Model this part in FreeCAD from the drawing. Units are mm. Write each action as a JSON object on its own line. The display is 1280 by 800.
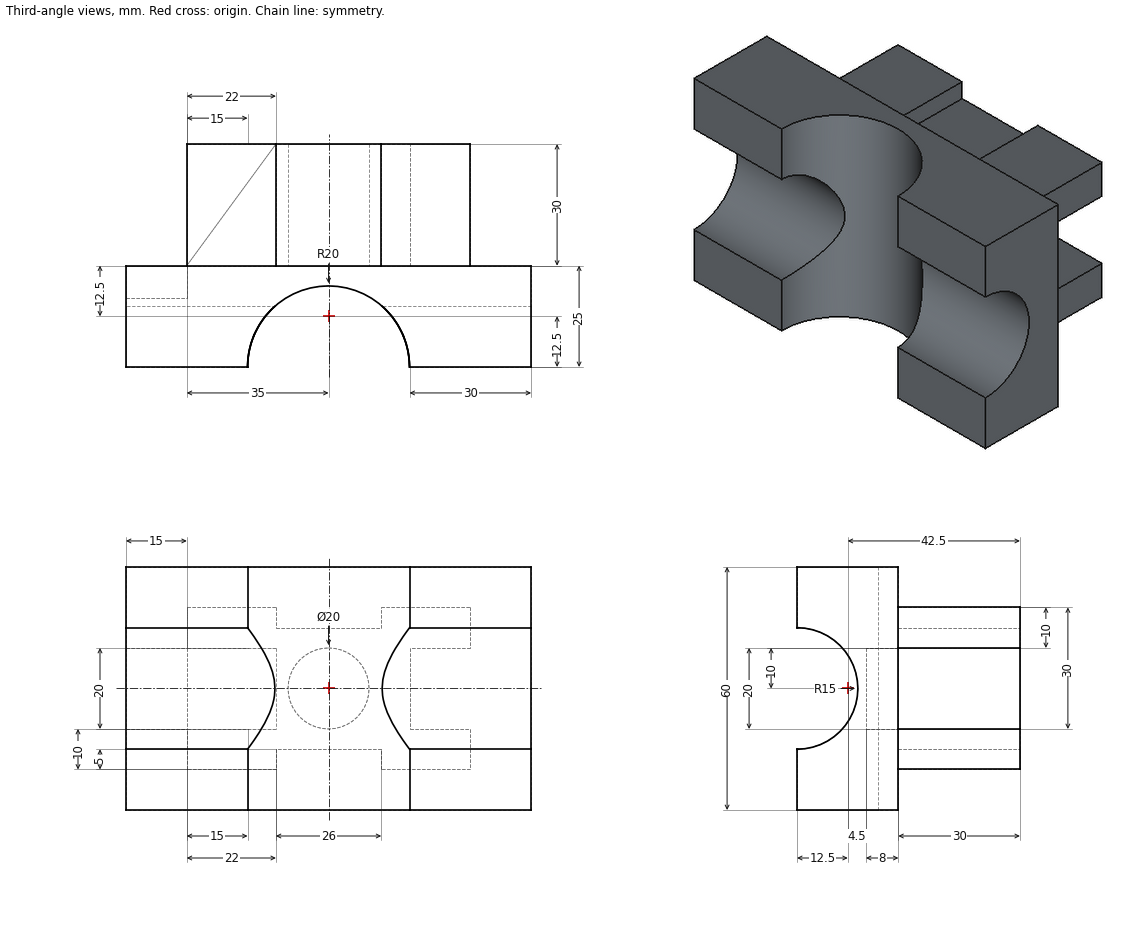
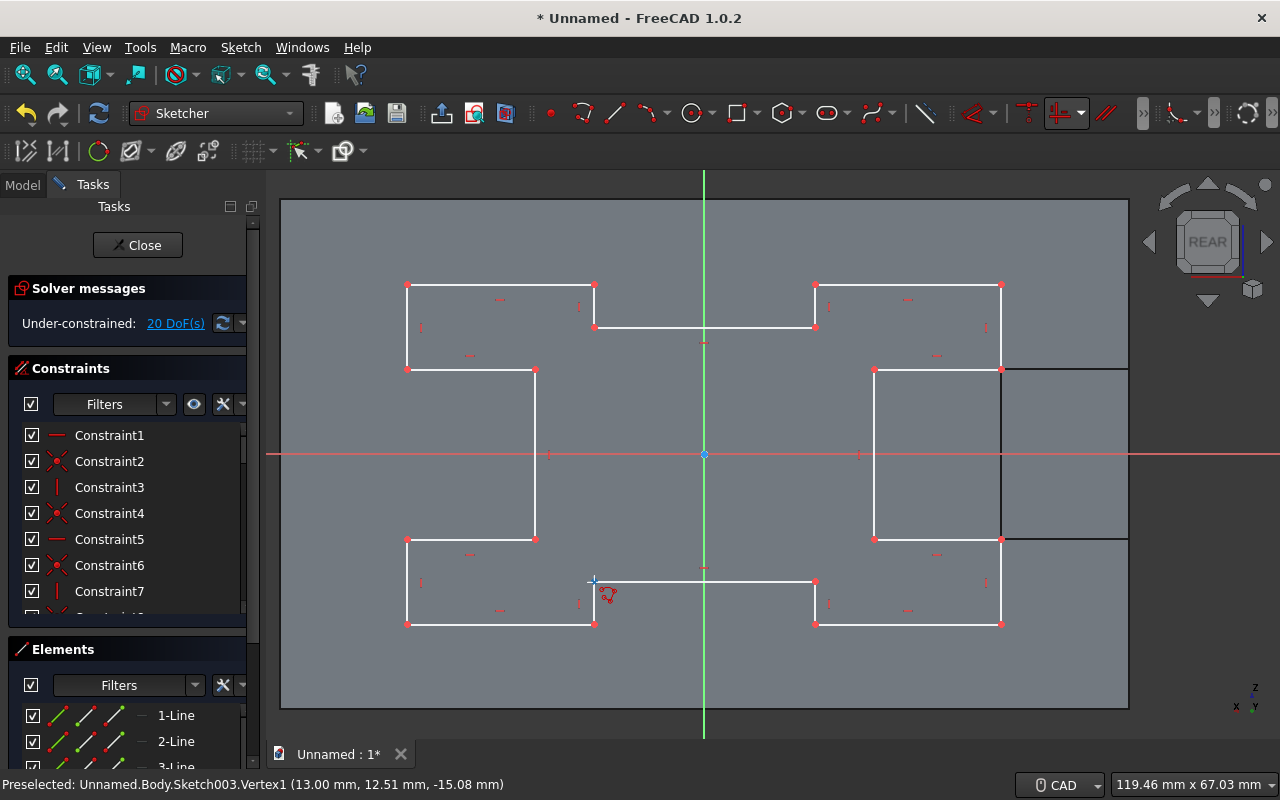
{"action": "key", "text": "g c"}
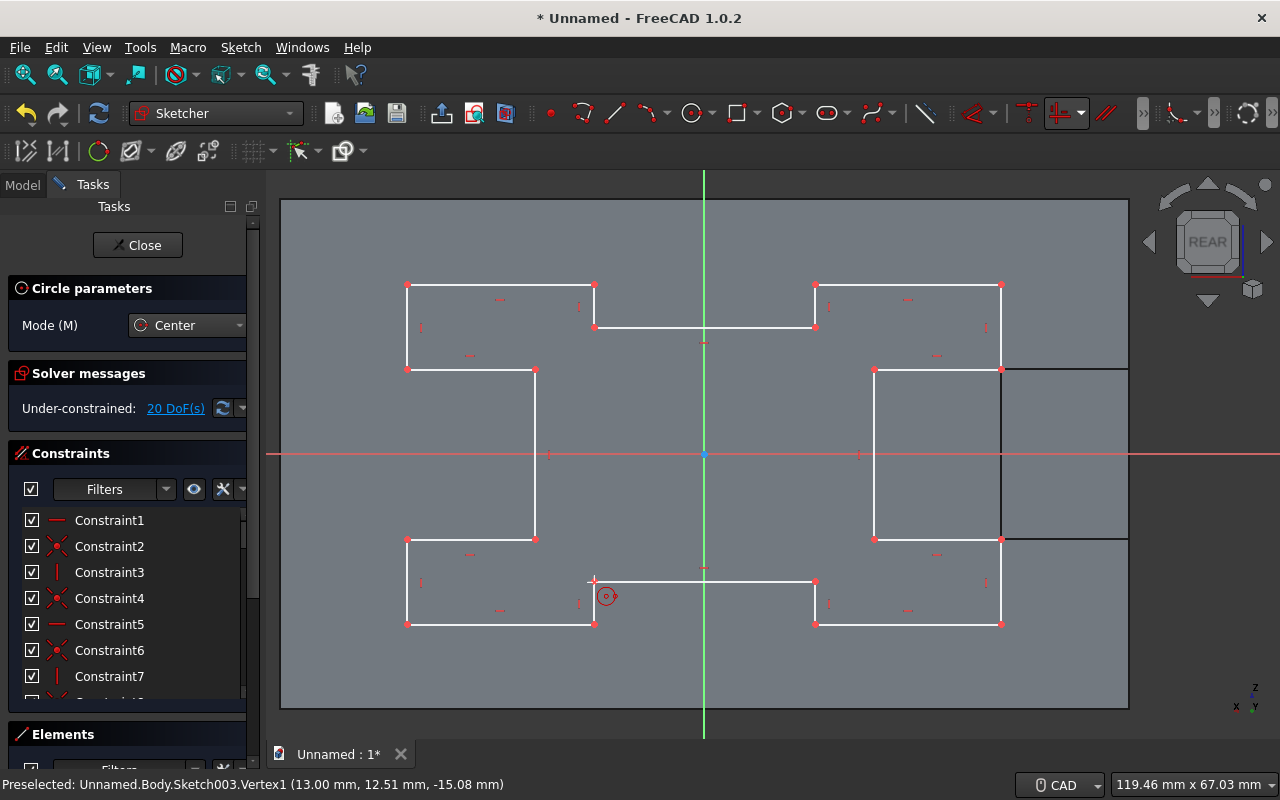
{"action": "left_click", "coordinate": [704, 454]}
{"action": "left_click", "coordinate": [764, 394]}
{"action": "key", "text": "Escape"}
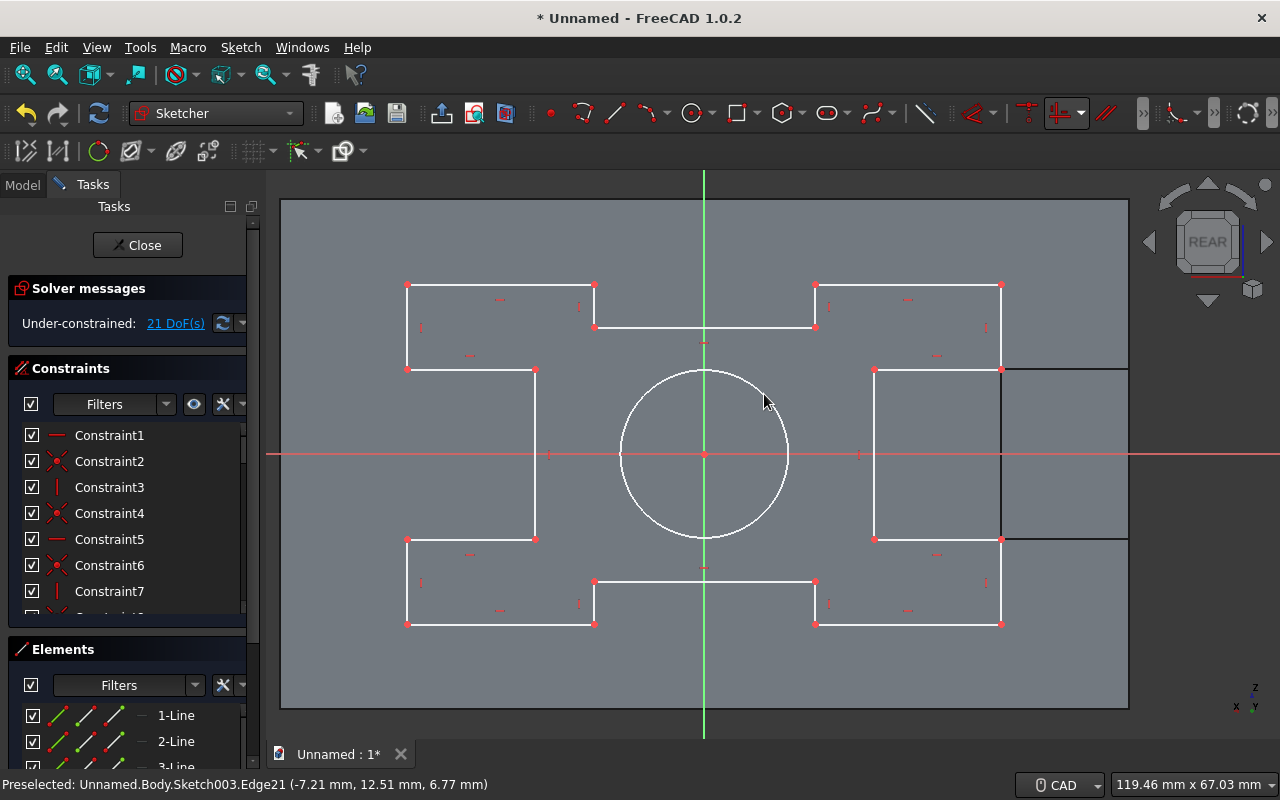
{"action": "left_click", "coordinate": [1001, 540]}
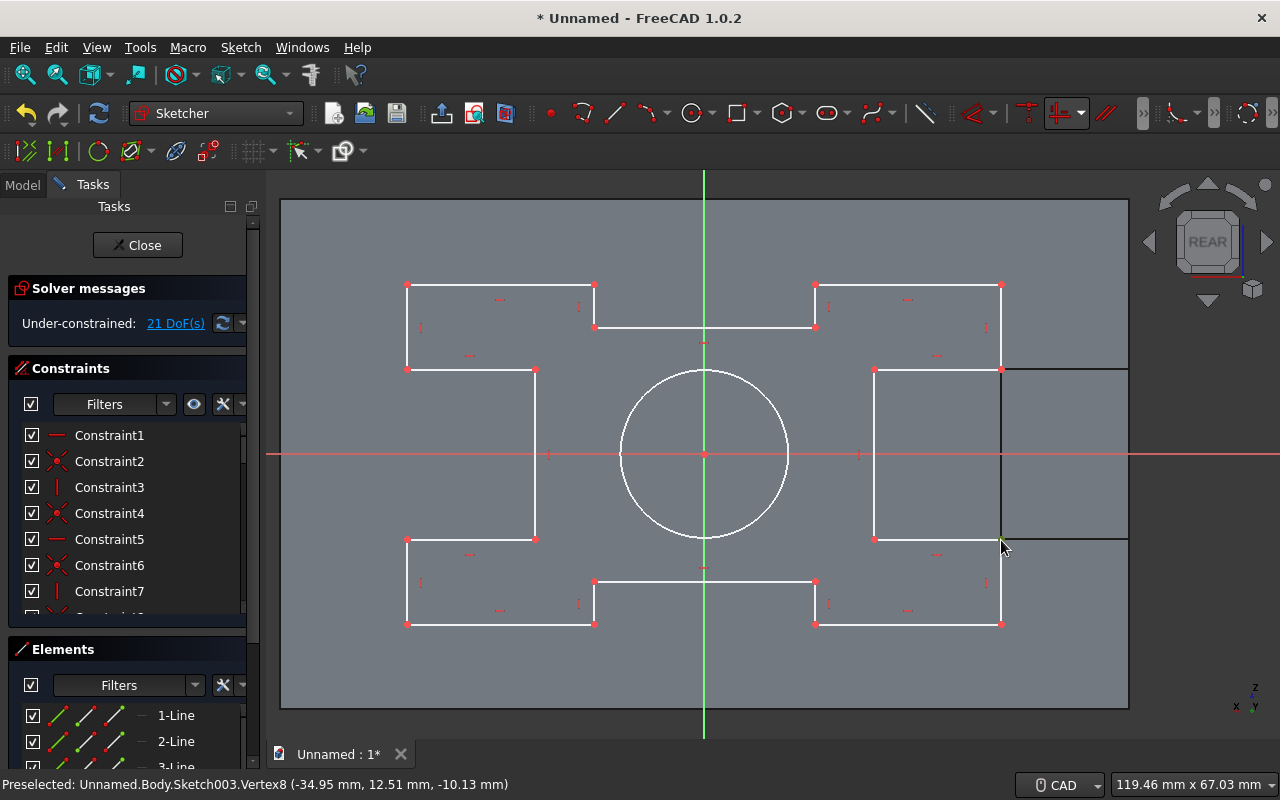
{"action": "left_click", "coordinate": [1001, 370]}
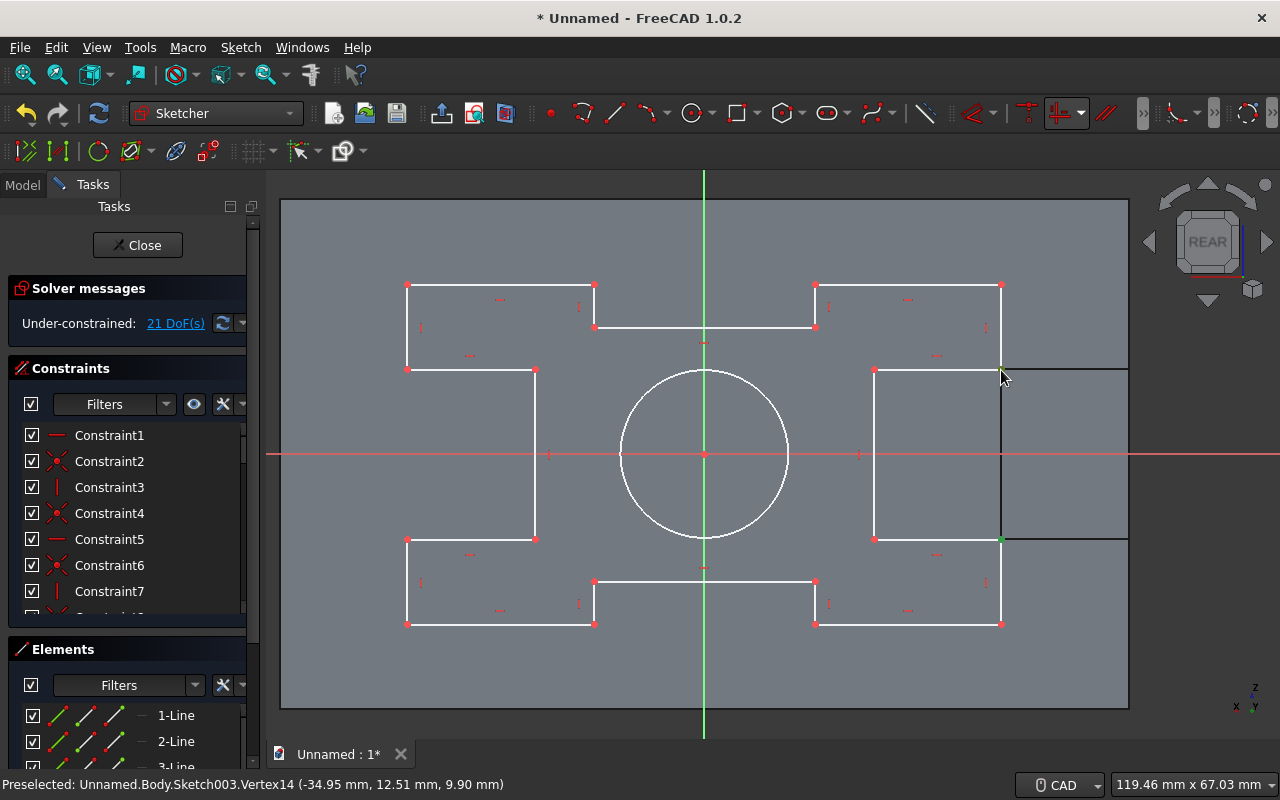
{"action": "left_click", "coordinate": [353, 454]}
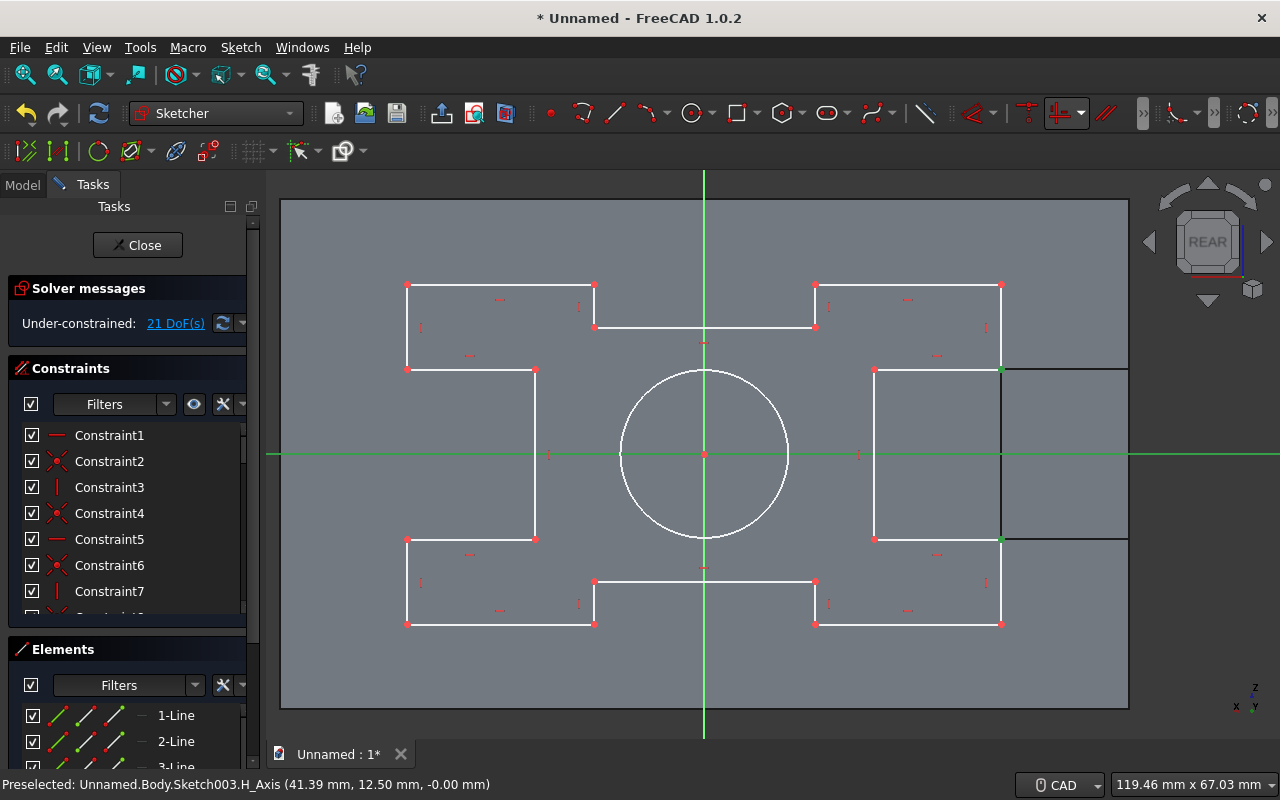
{"action": "key", "text": "s"}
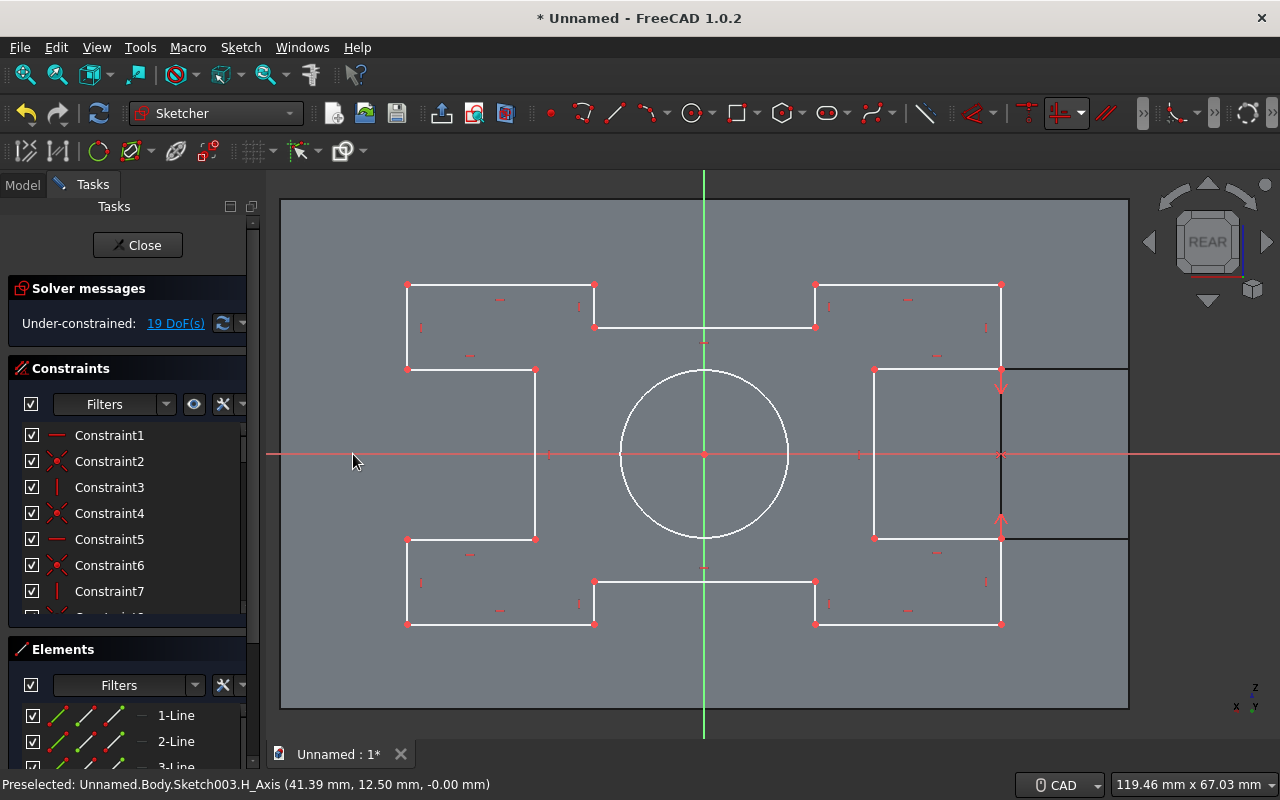
{"action": "left_click", "coordinate": [815, 625]}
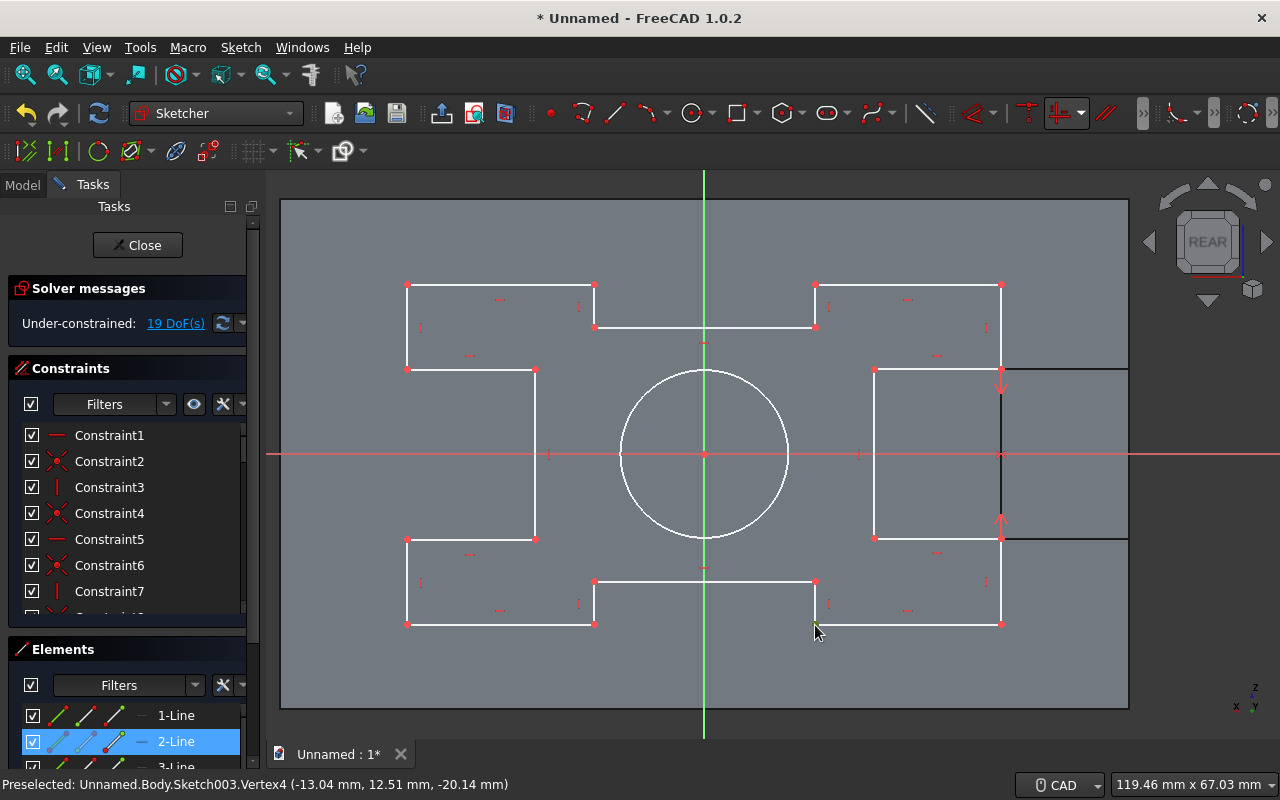
{"action": "left_click", "coordinate": [815, 285]}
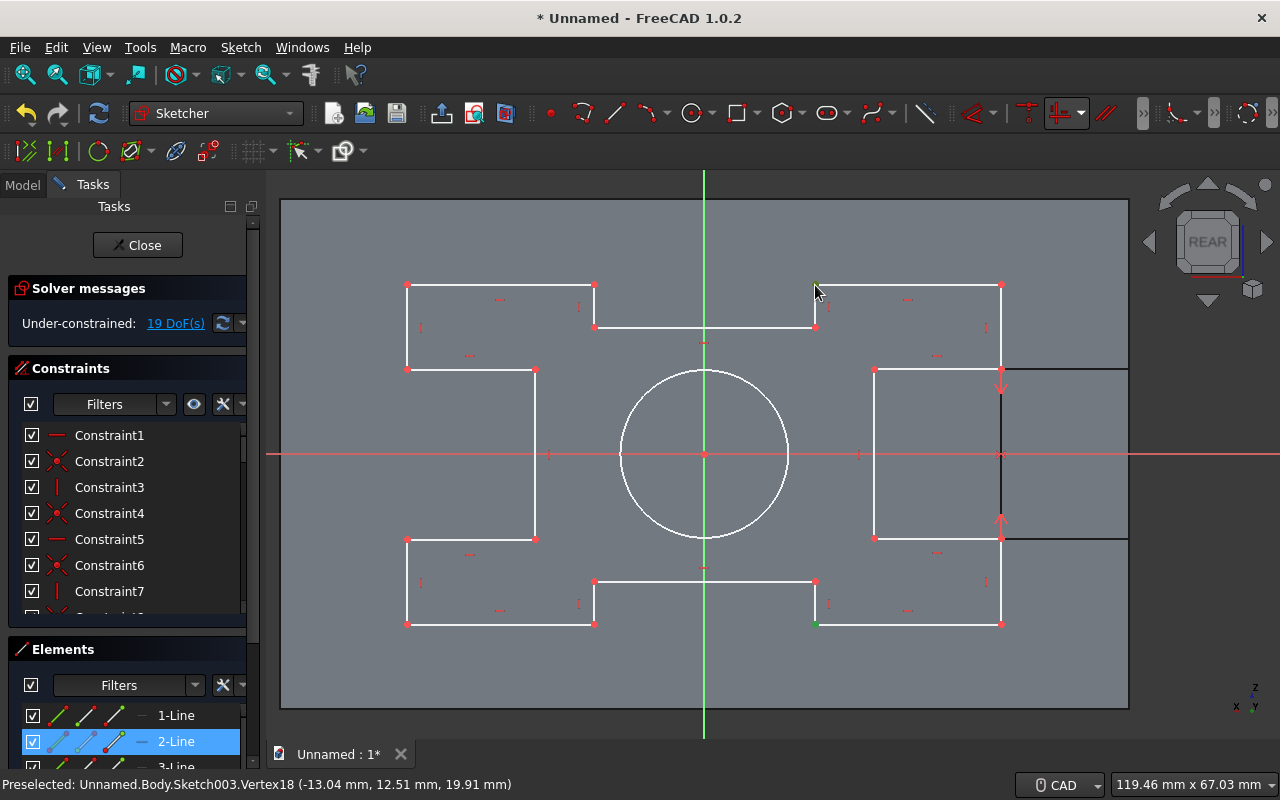
{"action": "left_click", "coordinate": [353, 454]}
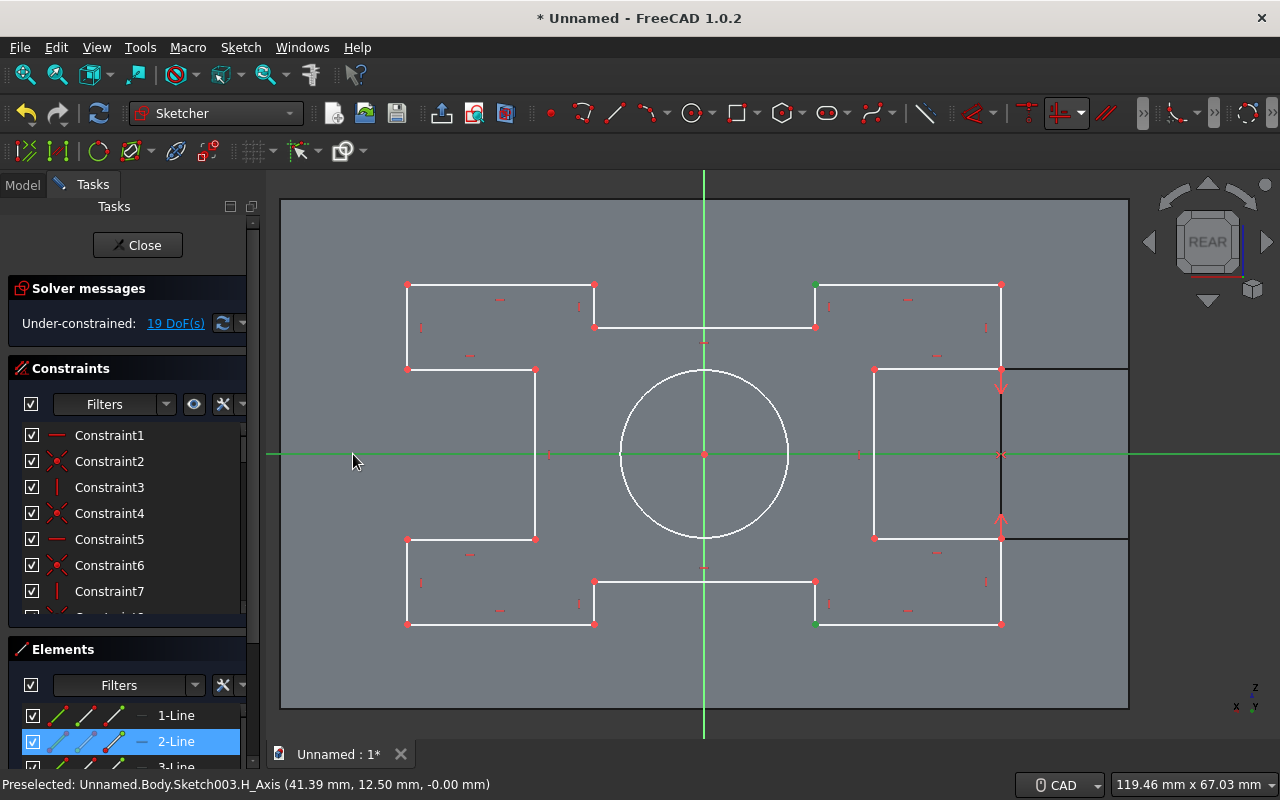
{"action": "key", "text": "s"}